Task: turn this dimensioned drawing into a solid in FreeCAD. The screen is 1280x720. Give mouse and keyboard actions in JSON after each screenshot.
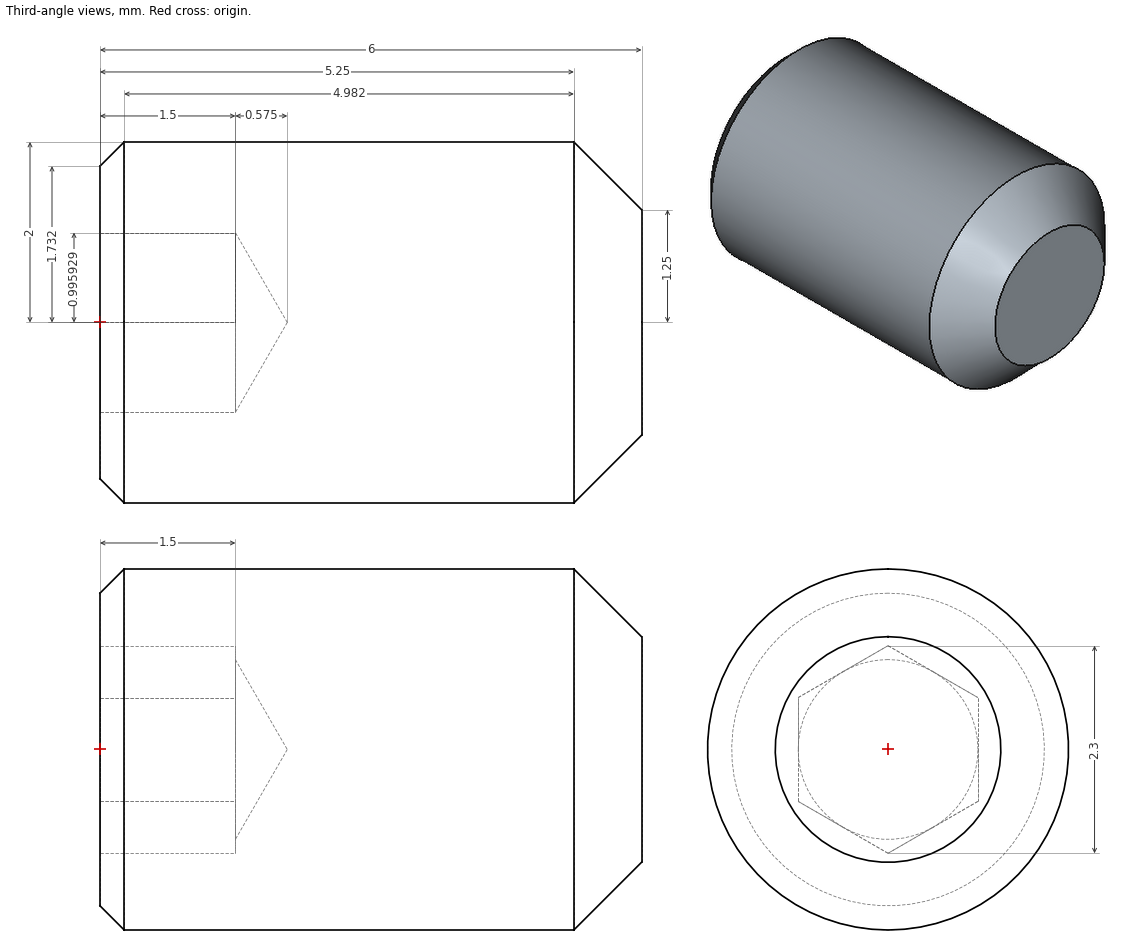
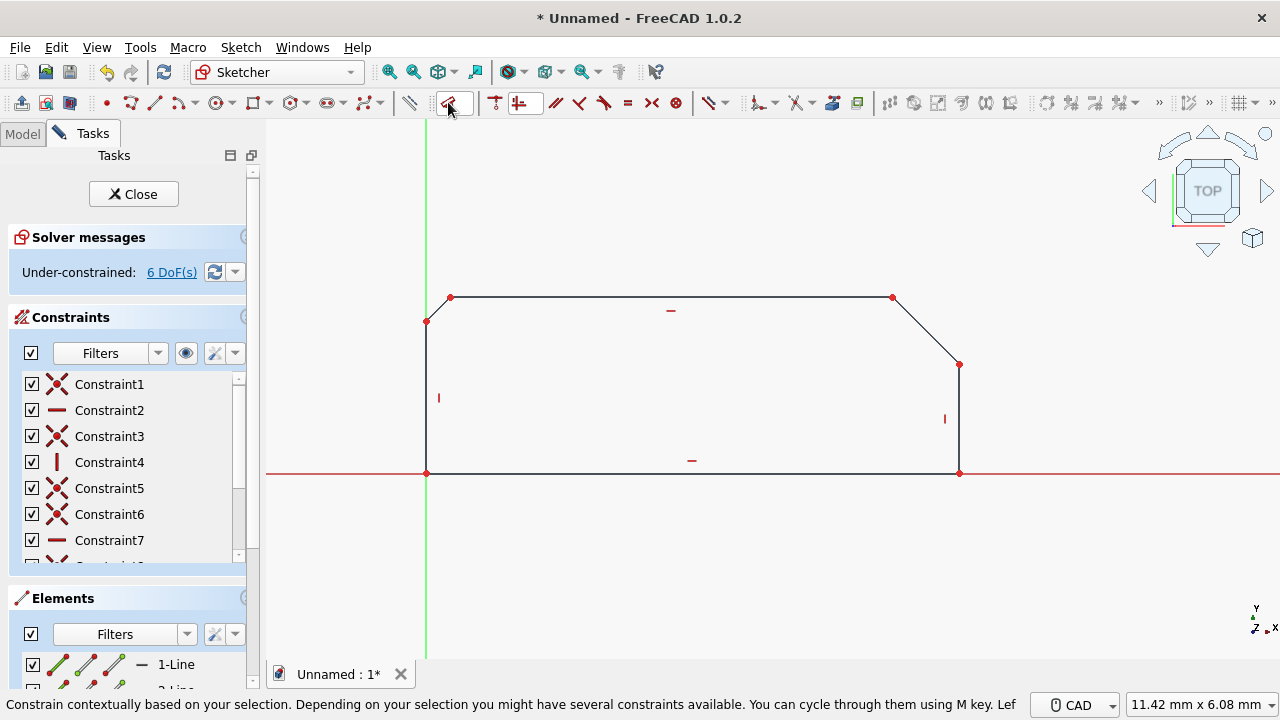
{"action": "left_click", "coordinate": [586, 474]}
{"action": "left_click", "coordinate": [693, 508]}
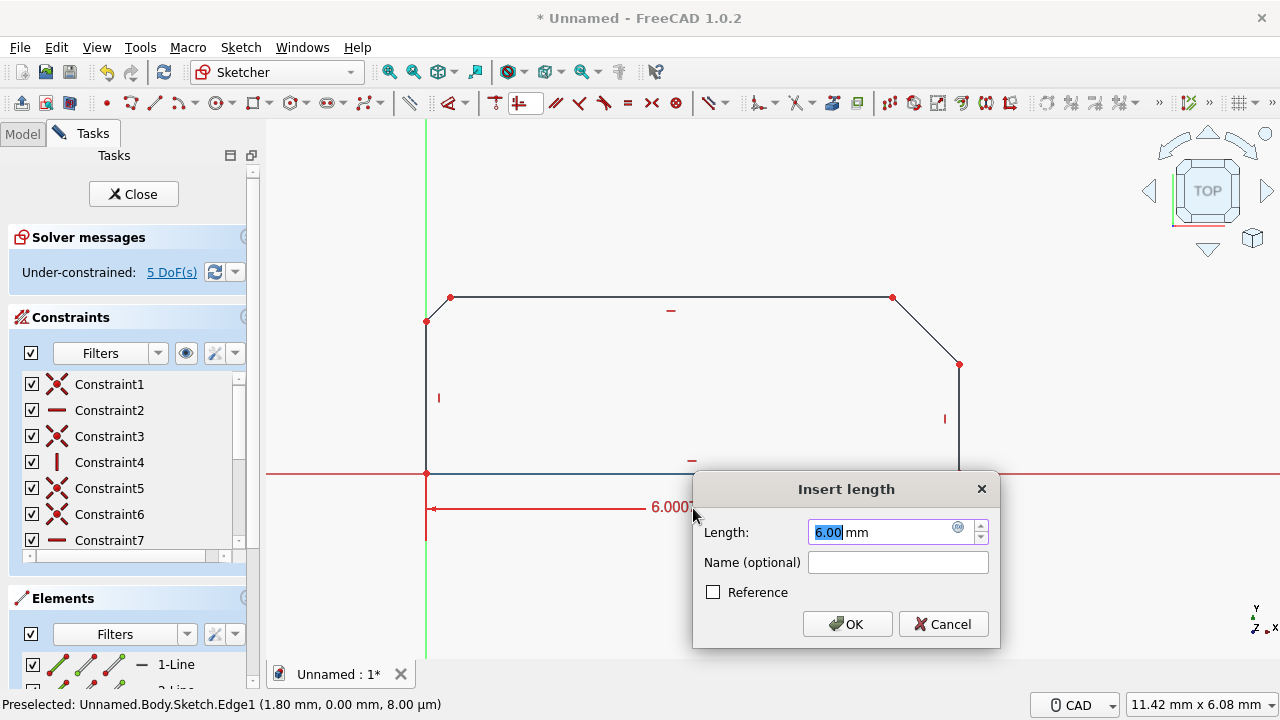
{"action": "type", "text": "6"}
{"action": "key", "text": "Return"}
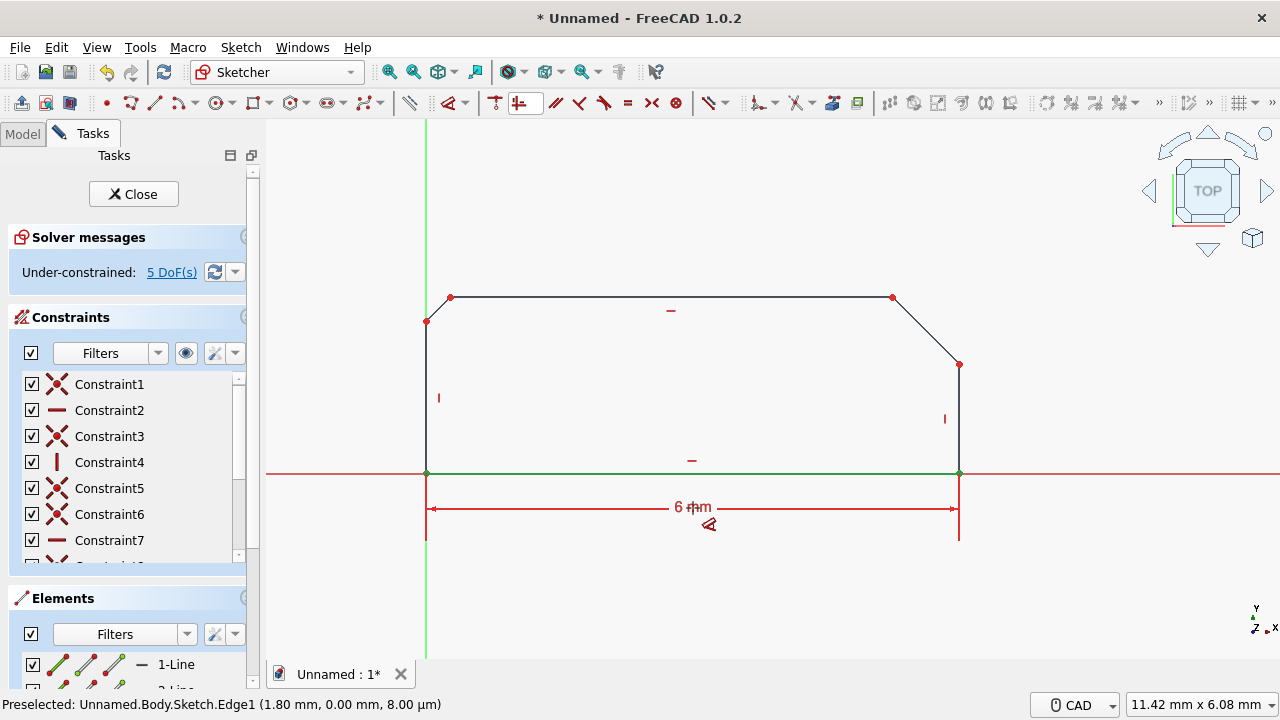
{"action": "left_click", "coordinate": [893, 297]}
{"action": "left_click", "coordinate": [392, 386]}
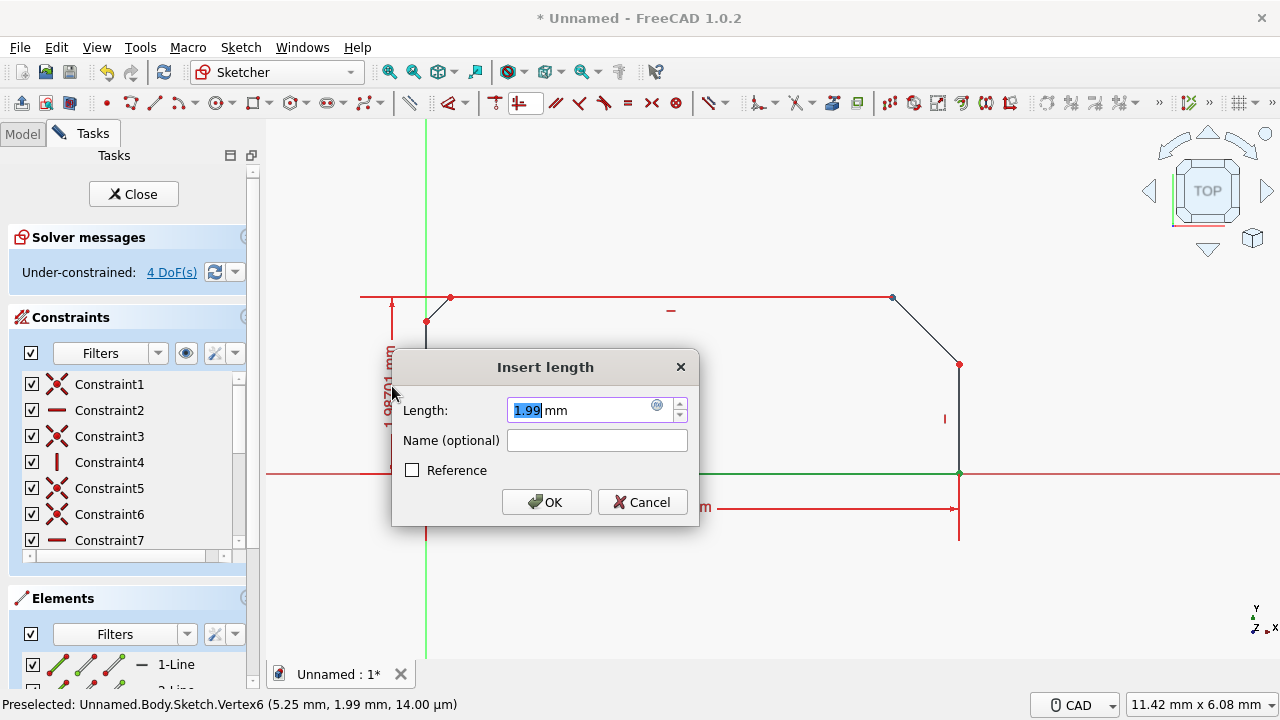
{"action": "type", "text": "2"}
{"action": "key", "text": "Return"}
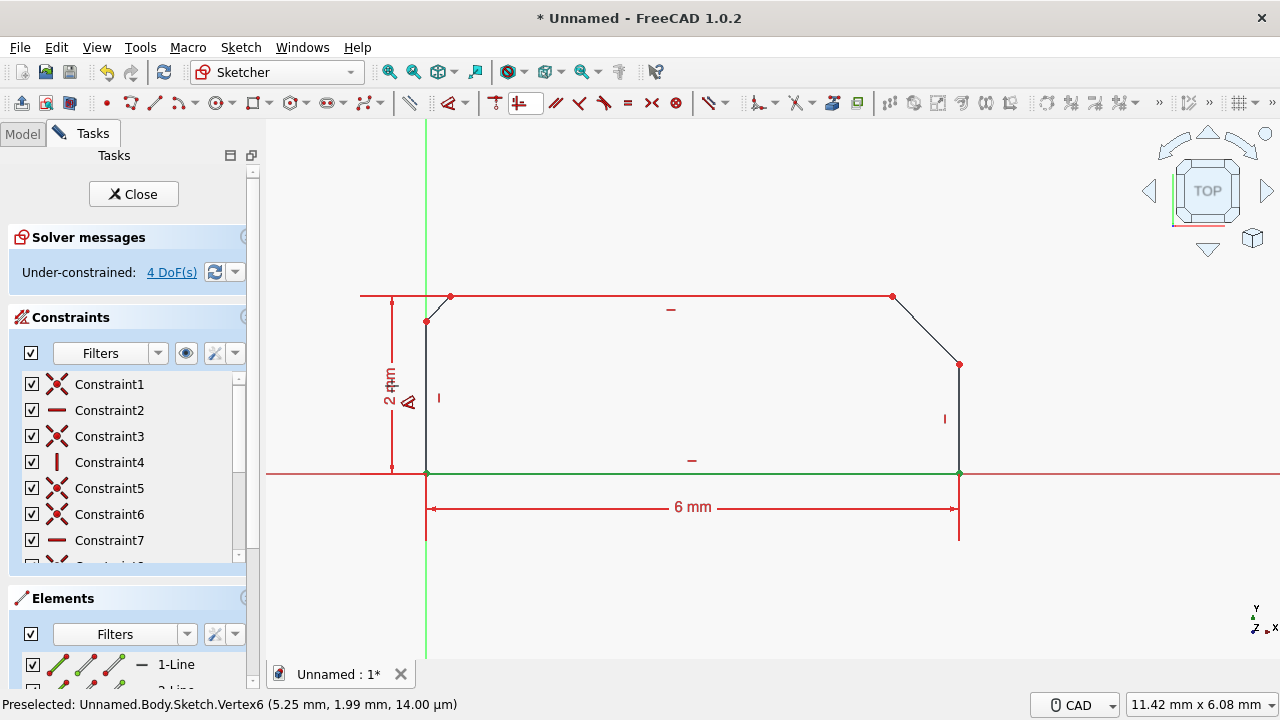
{"action": "left_click", "coordinate": [959, 441]}
{"action": "left_click", "coordinate": [993, 419]}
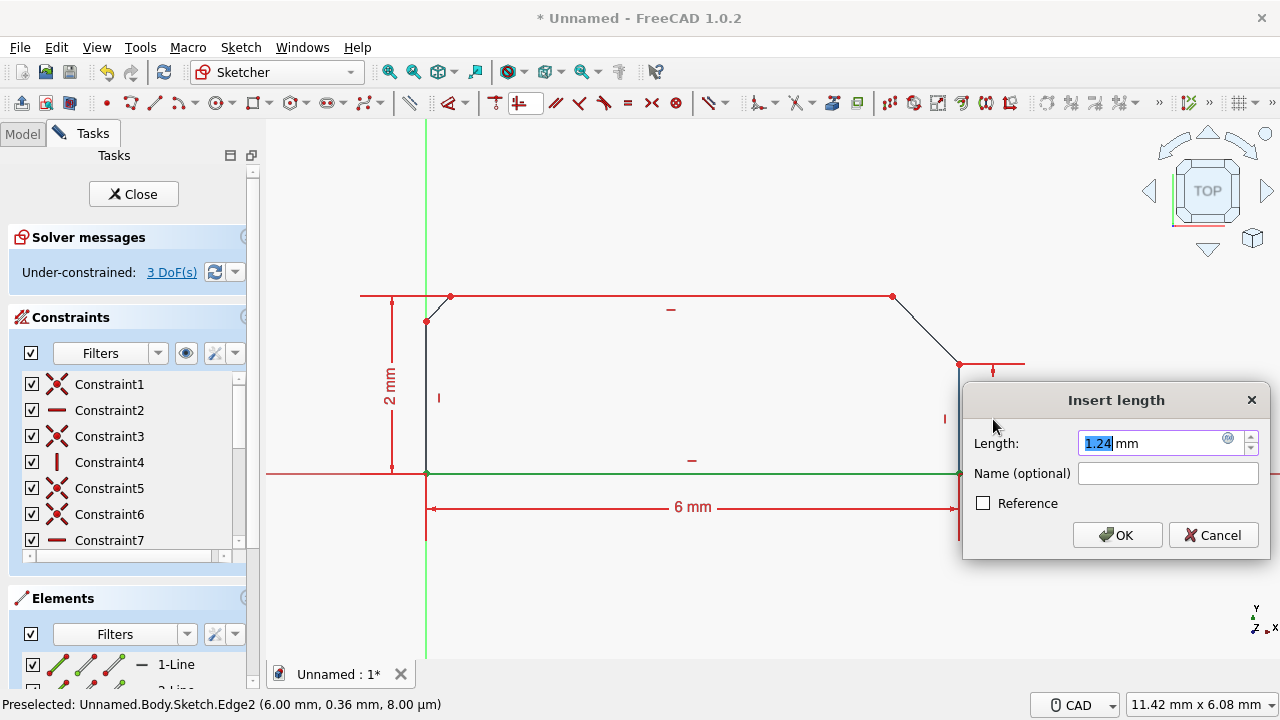
{"action": "type", "text": "1.25"}
{"action": "key", "text": "Return"}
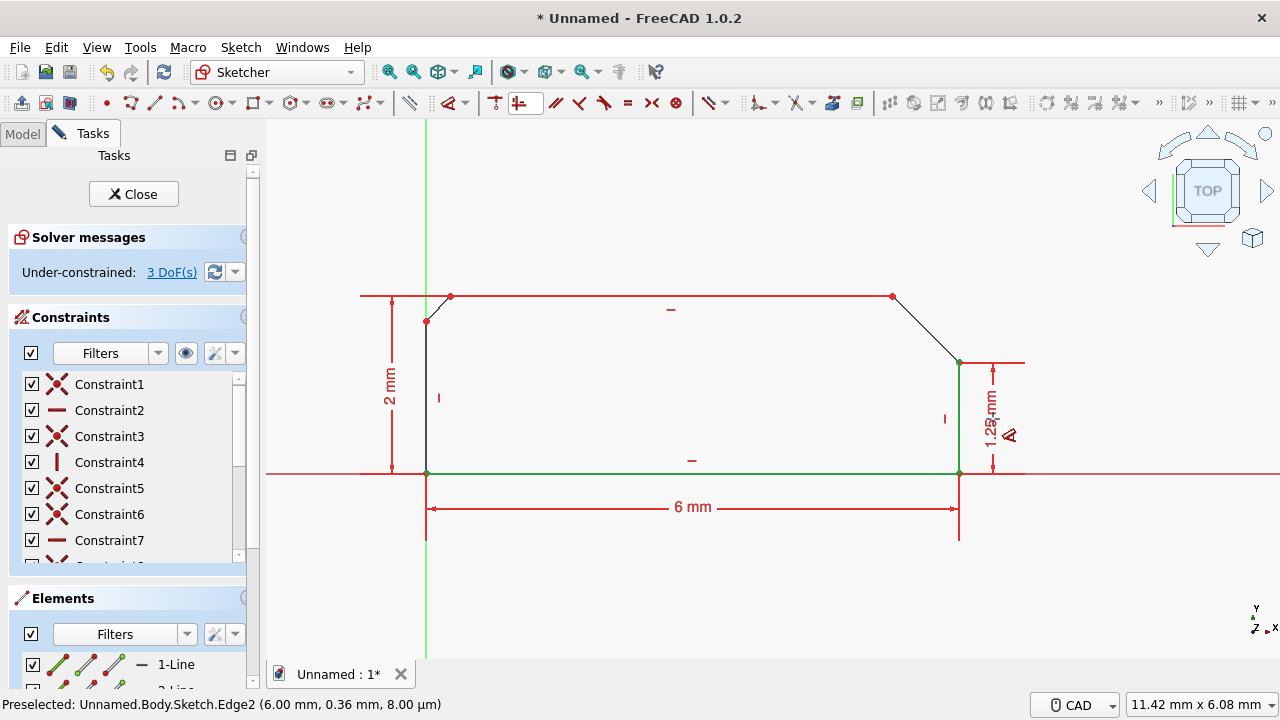
{"action": "left_click", "coordinate": [760, 296]}
{"action": "left_click", "coordinate": [671, 262]}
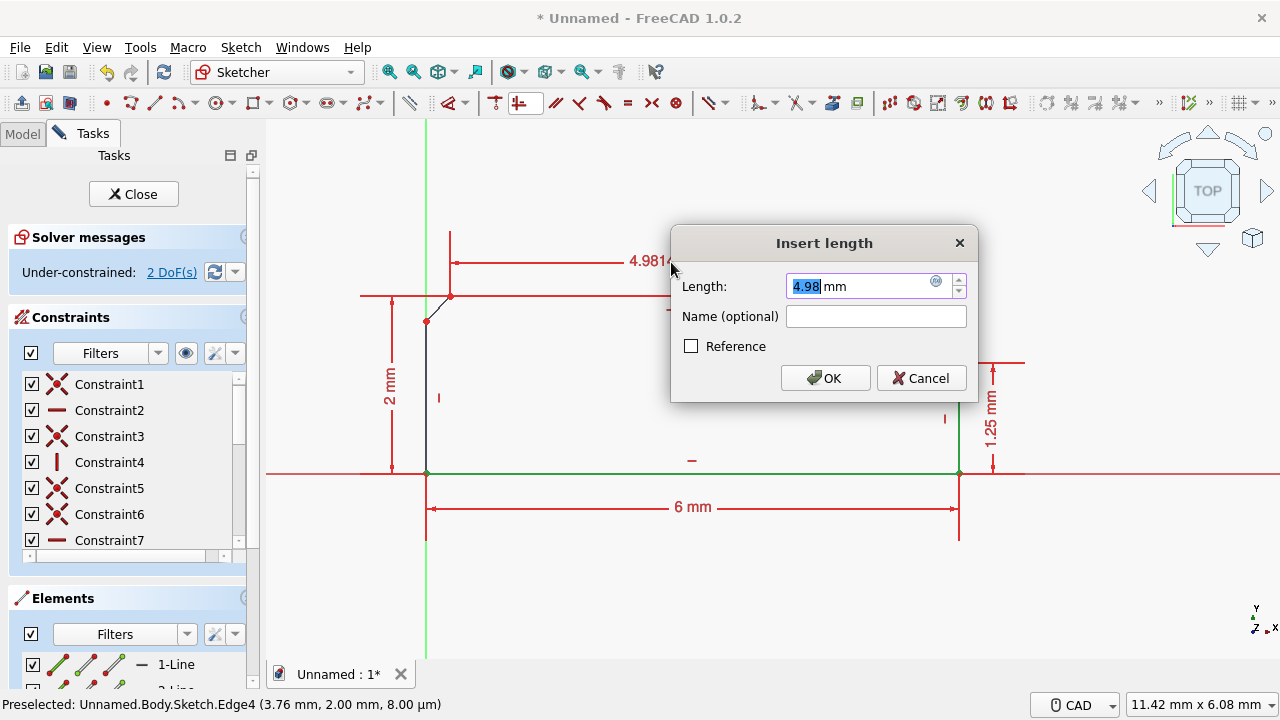
{"action": "type", "text": "4.982"}
{"action": "key", "text": "Return"}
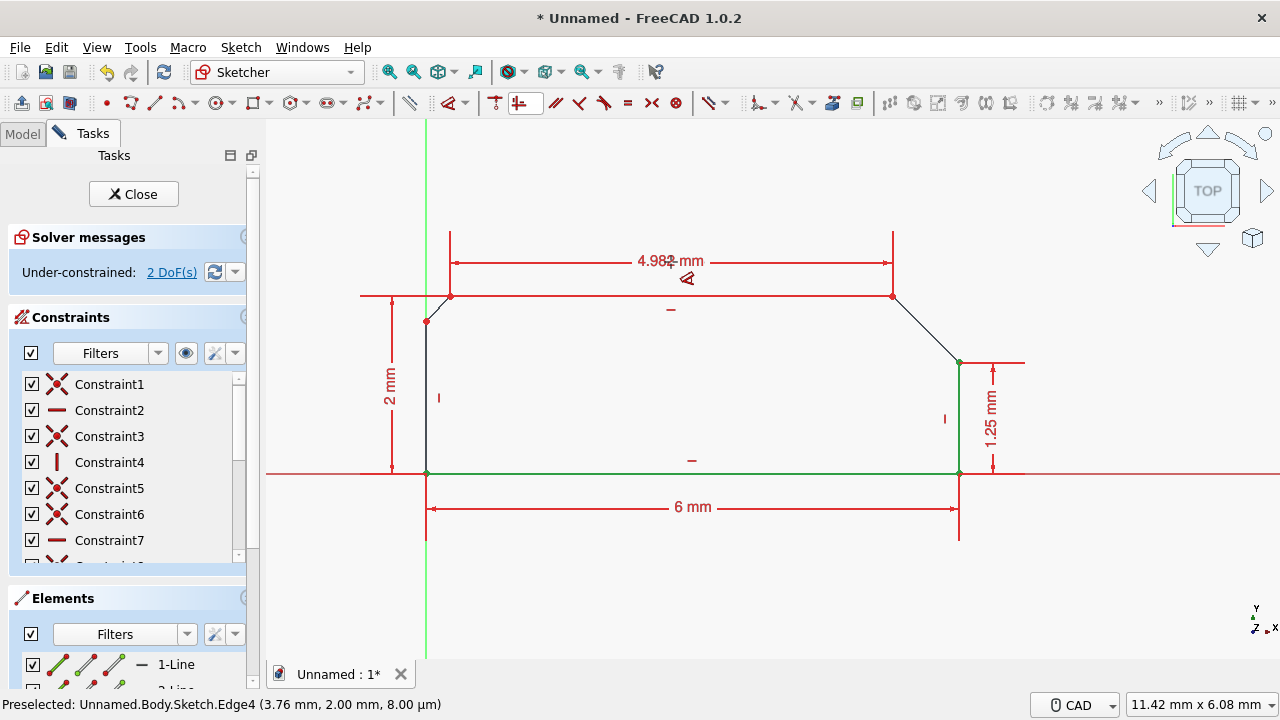
{"action": "left_click", "coordinate": [426, 367]}
{"action": "left_click", "coordinate": [392, 362]}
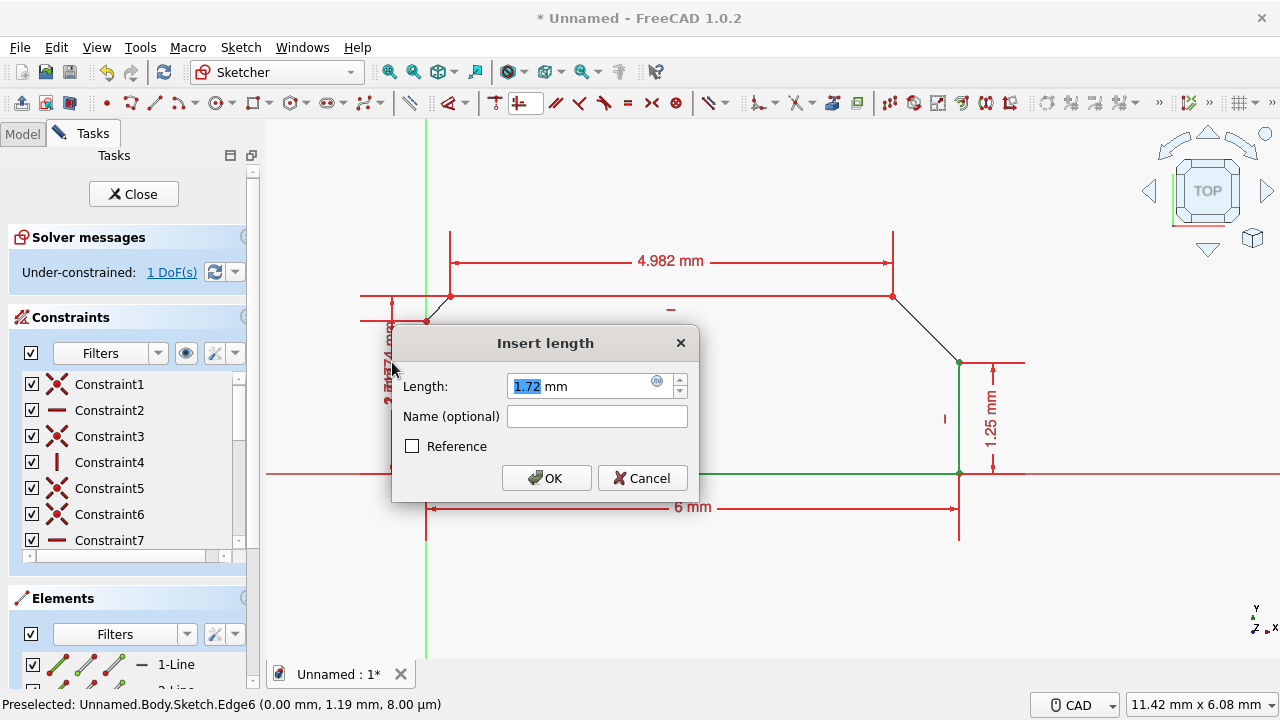
{"action": "type", "text": "1.732"}
{"action": "key", "text": "Return"}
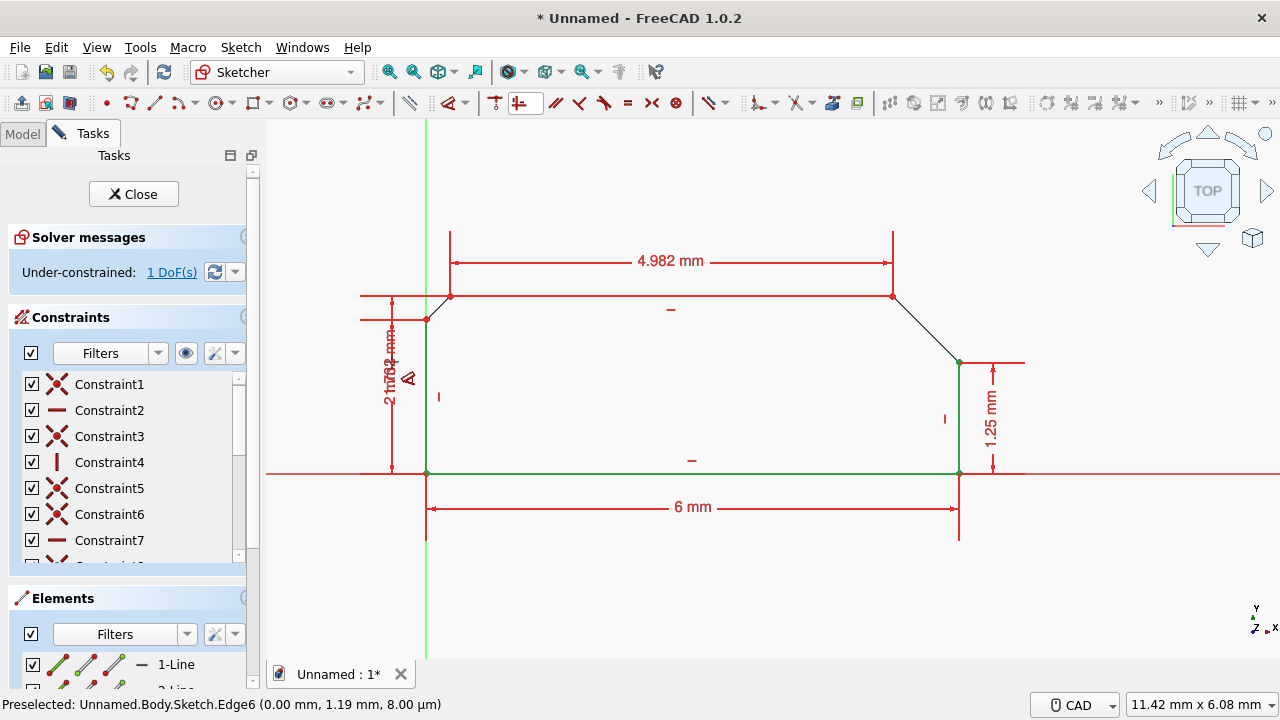
{"action": "left_click", "coordinate": [893, 296]}
{"action": "left_click", "coordinate": [552, 508]}